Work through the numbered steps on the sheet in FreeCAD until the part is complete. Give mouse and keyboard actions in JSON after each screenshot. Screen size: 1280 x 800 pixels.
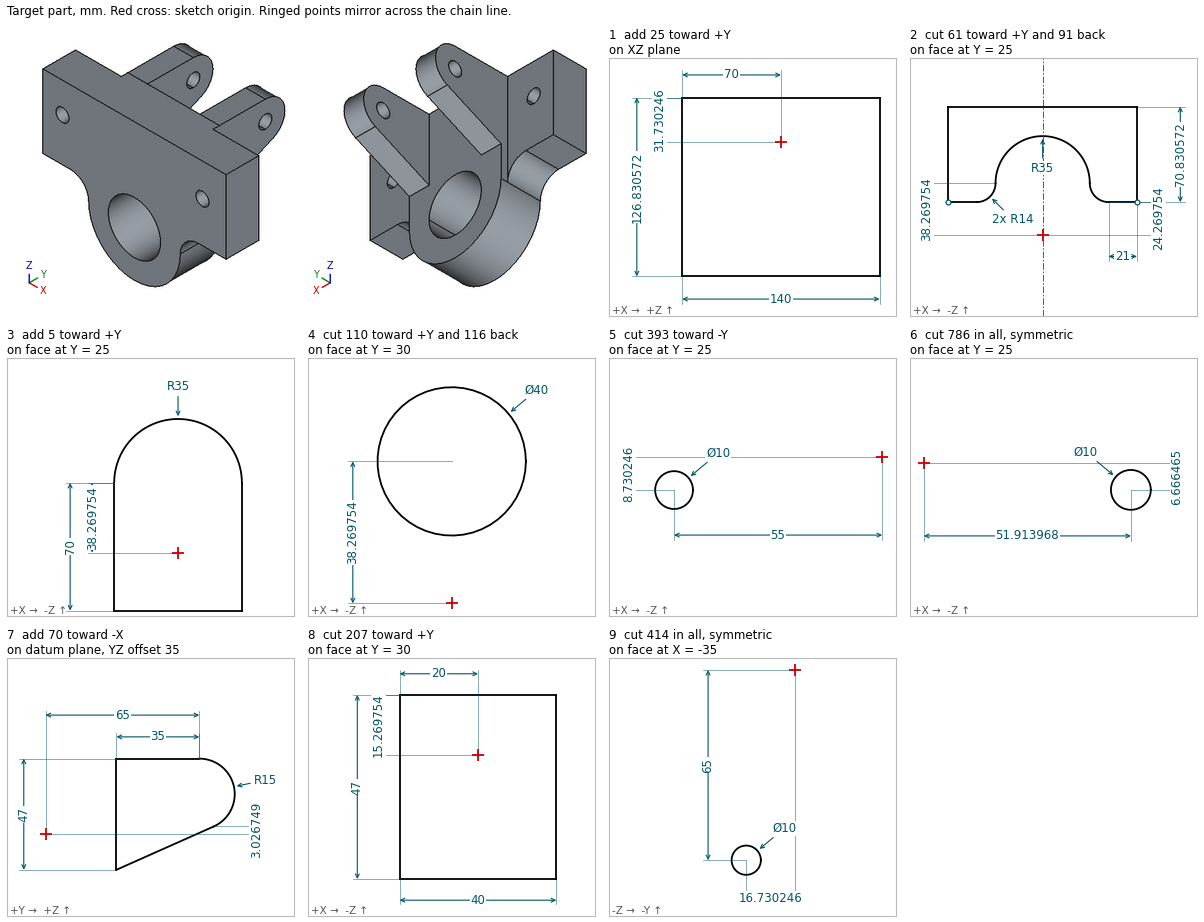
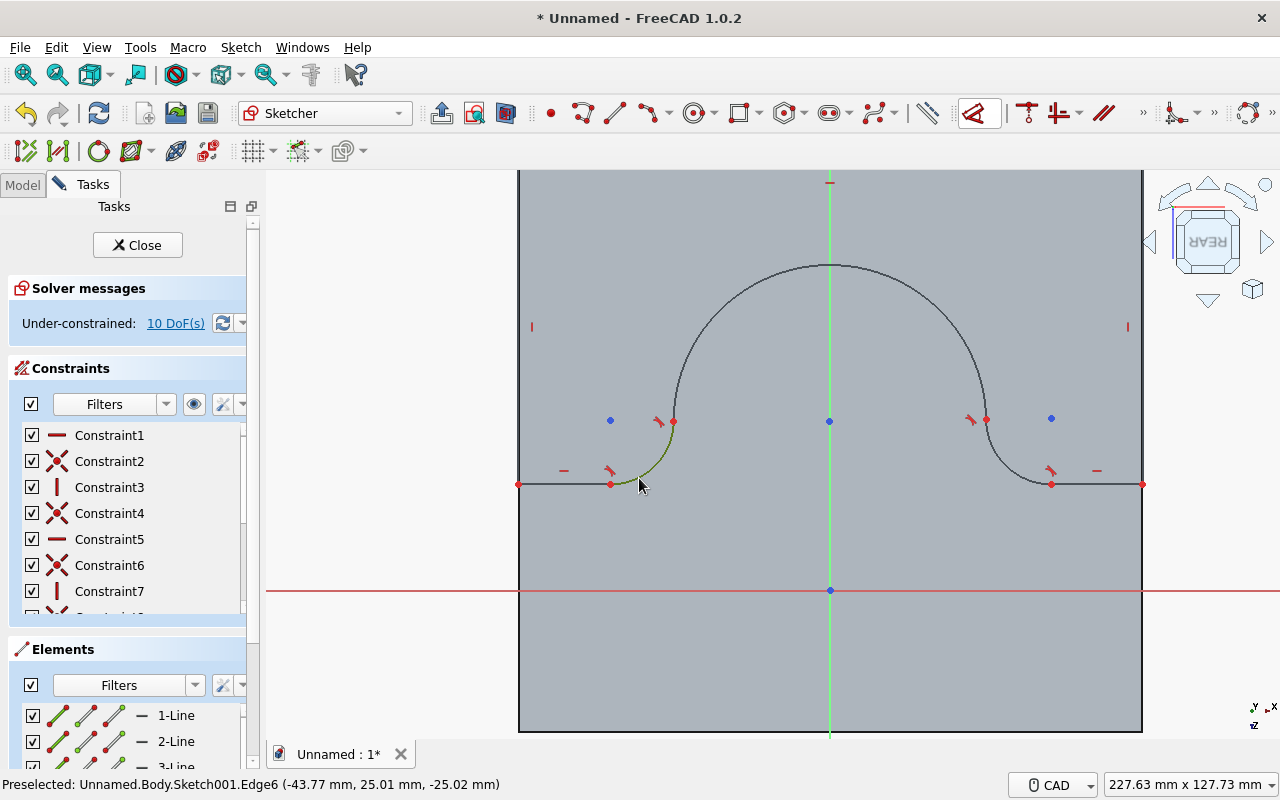
{"action": "left_click", "coordinate": [993, 449]}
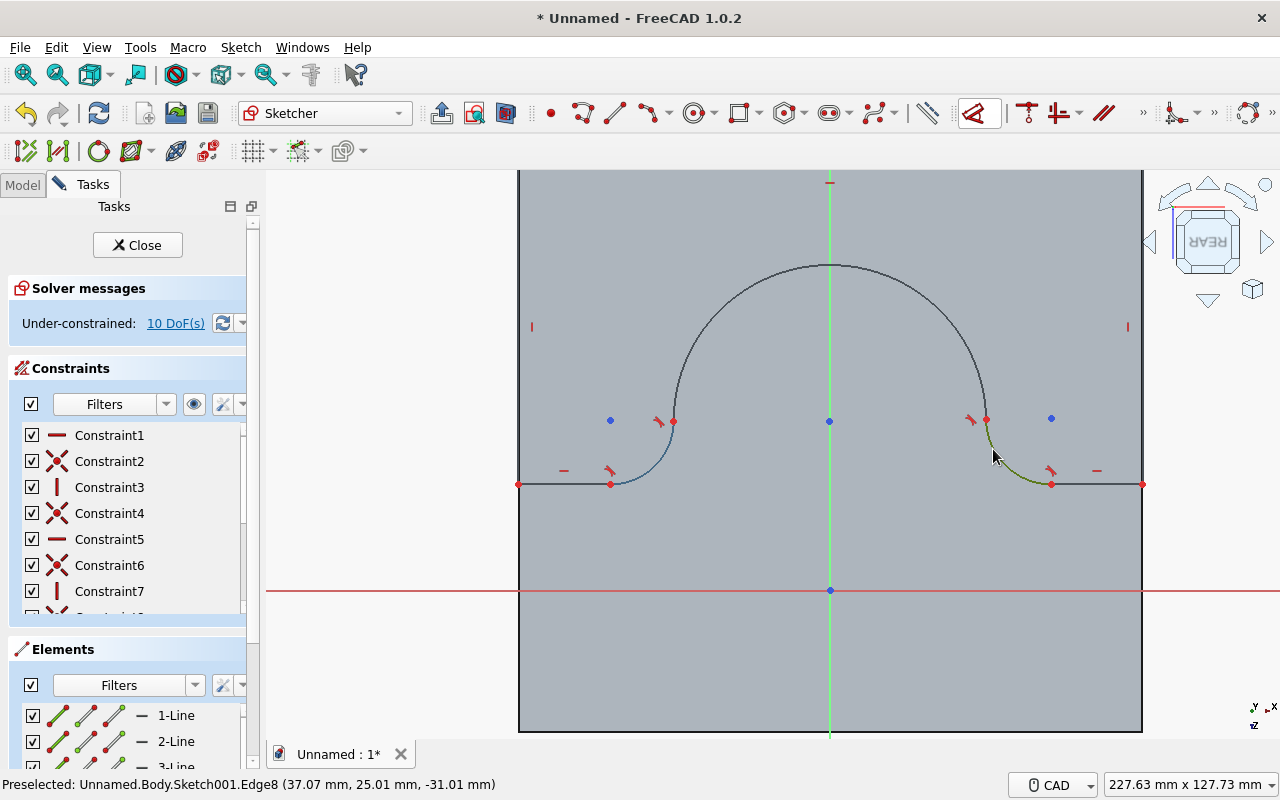
{"action": "key", "text": "e"}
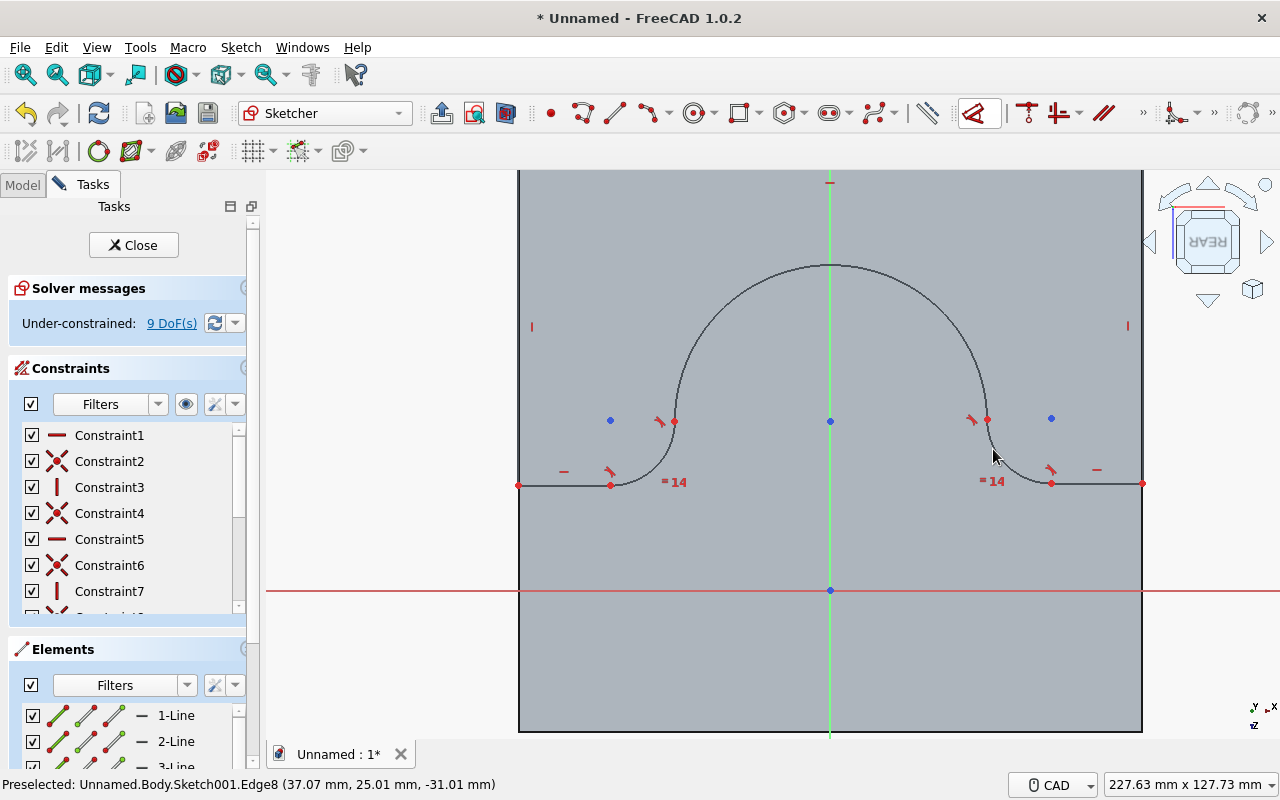
{"action": "left_click", "coordinate": [831, 421]}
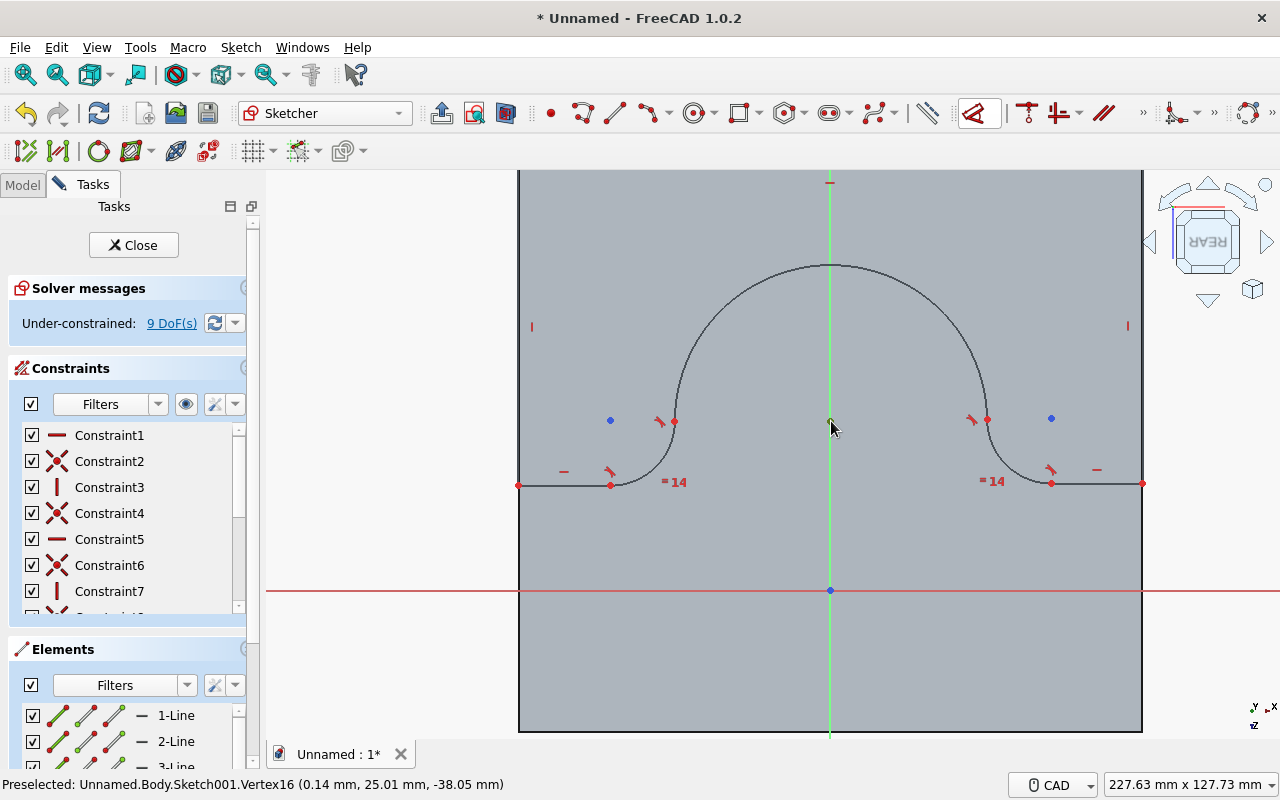
{"action": "left_click", "coordinate": [830, 674]}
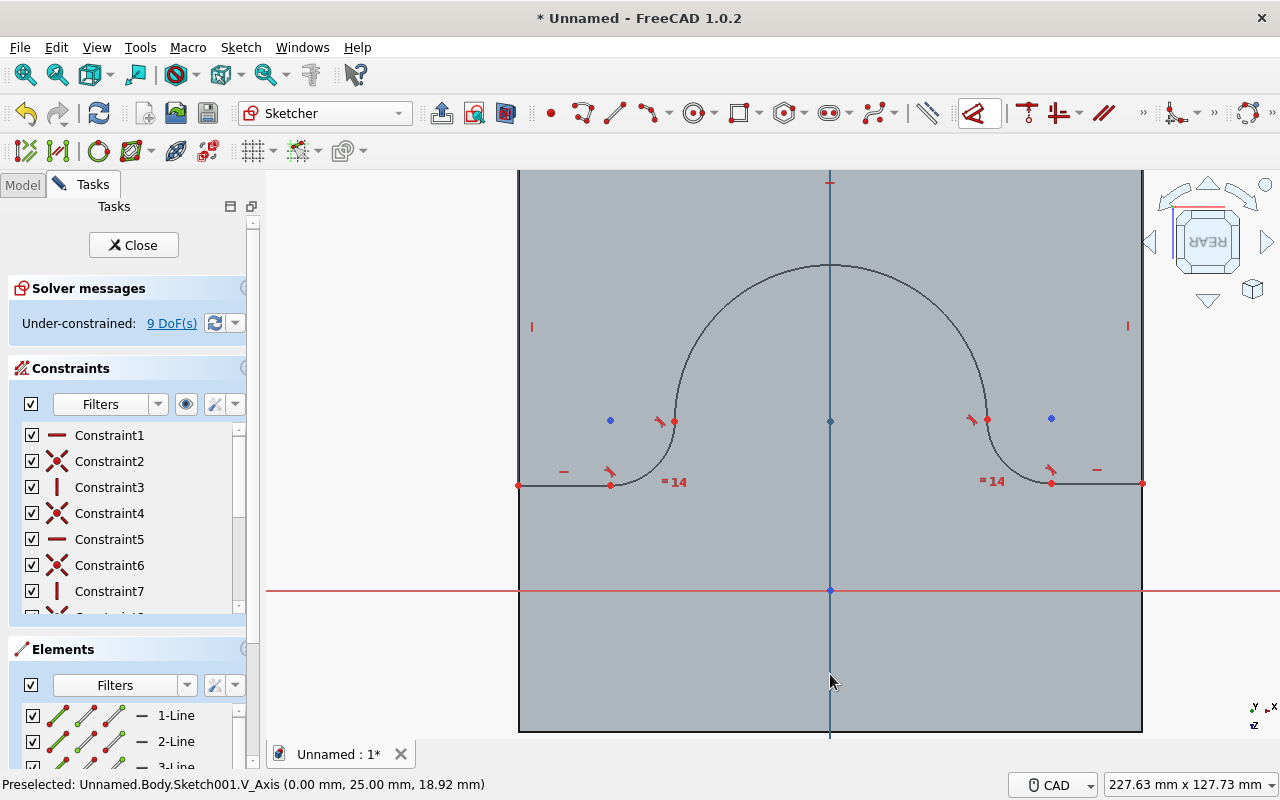
{"action": "left_click", "coordinate": [1028, 114]}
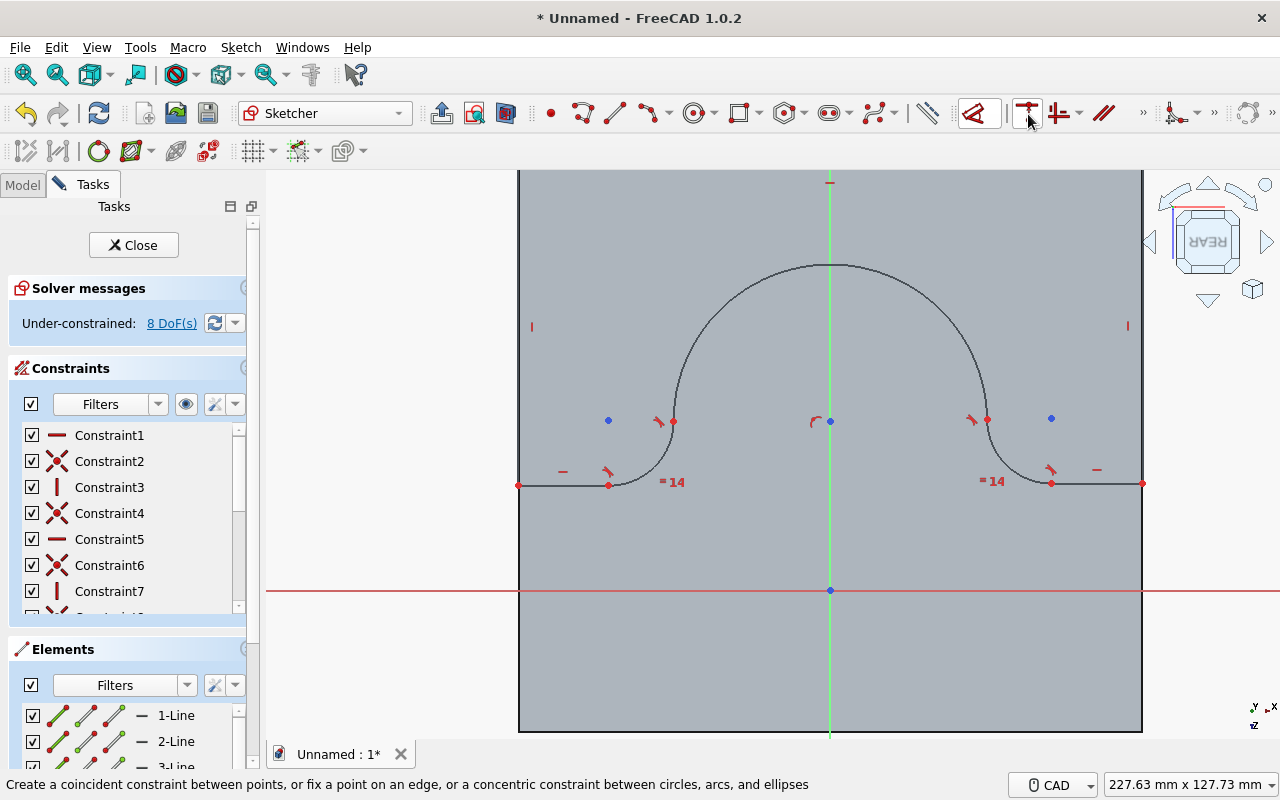
{"action": "scroll", "coordinate": [294, 711], "scroll_direction": "down", "scroll_amount": 1}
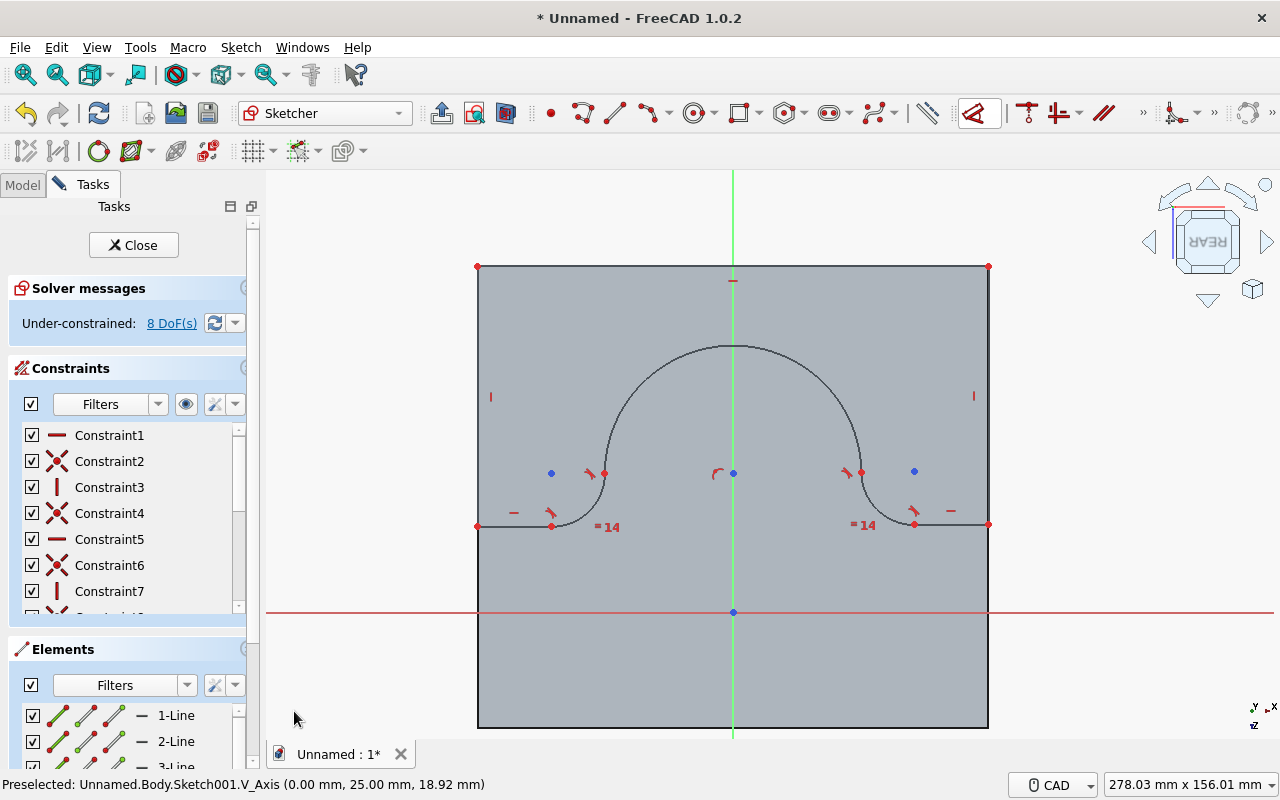
{"action": "left_click", "coordinate": [989, 525]}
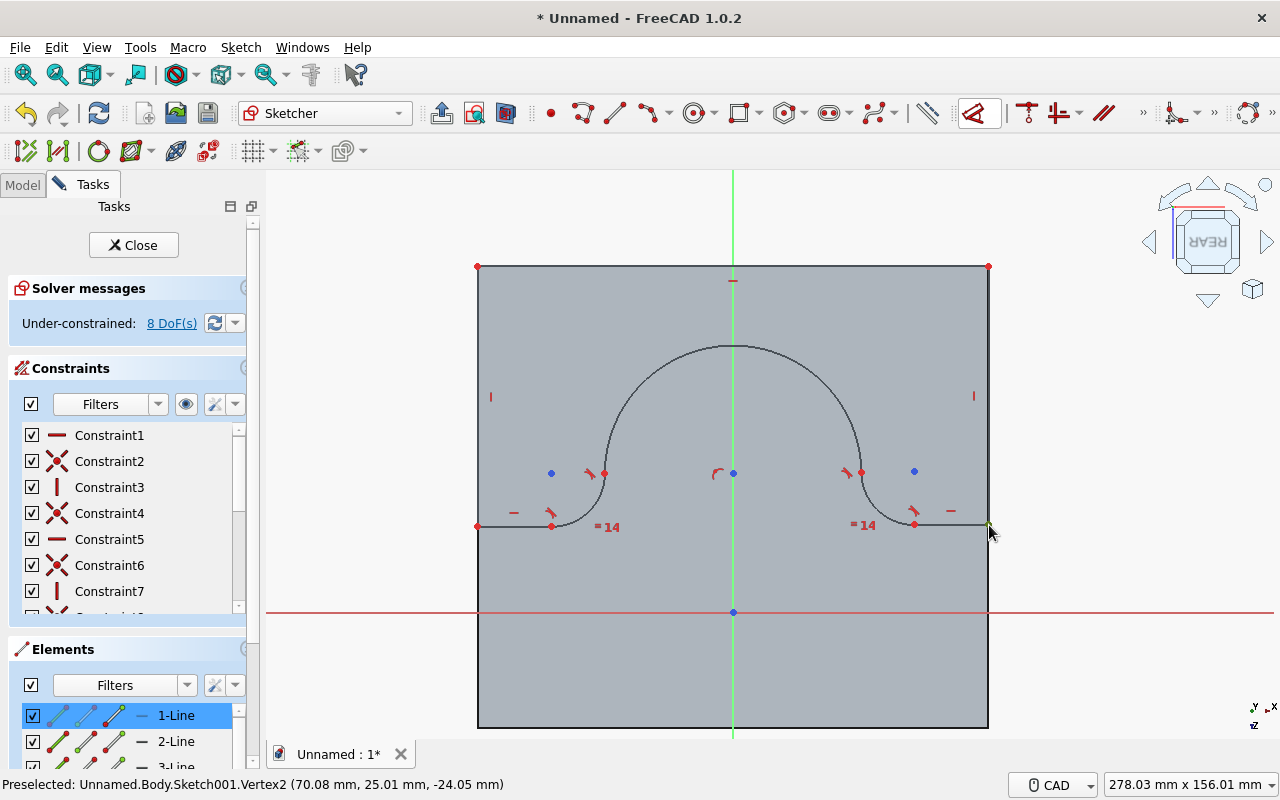
{"action": "left_click", "coordinate": [478, 527]}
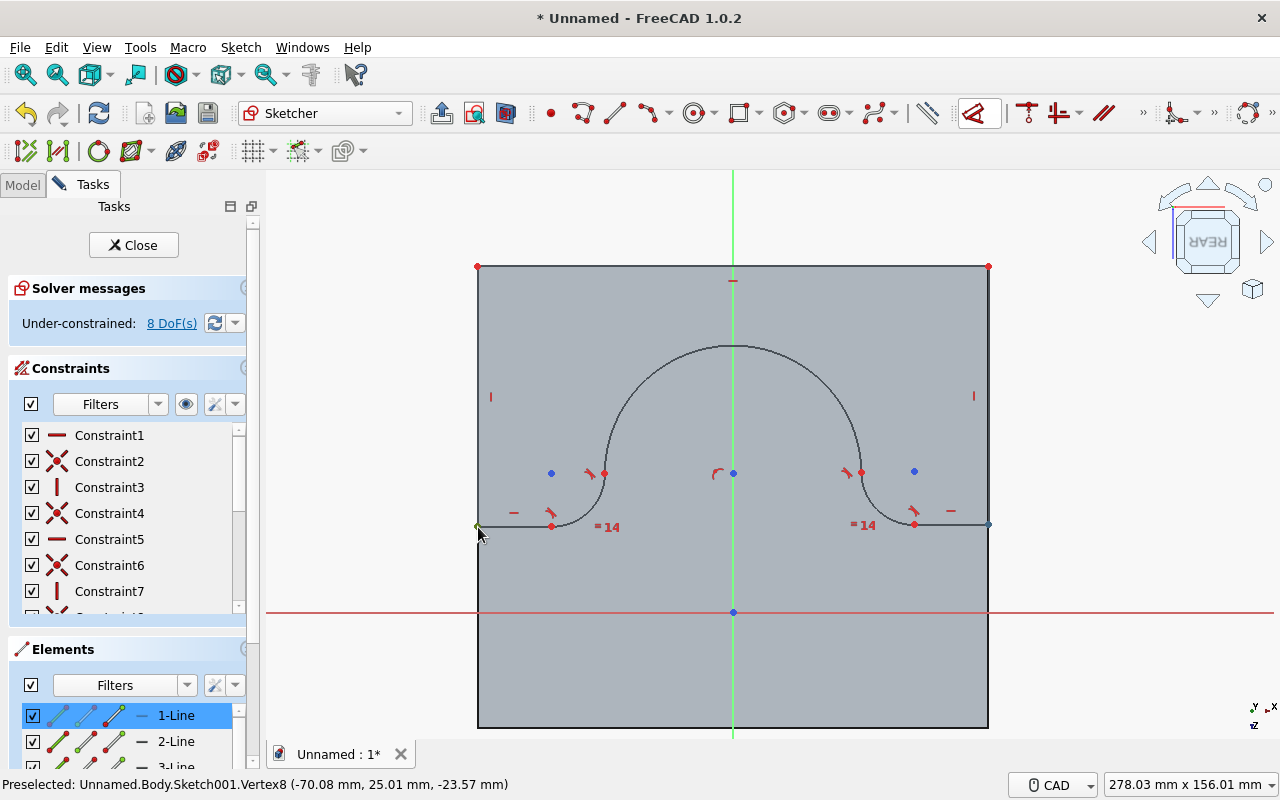
{"action": "left_click", "coordinate": [733, 674]}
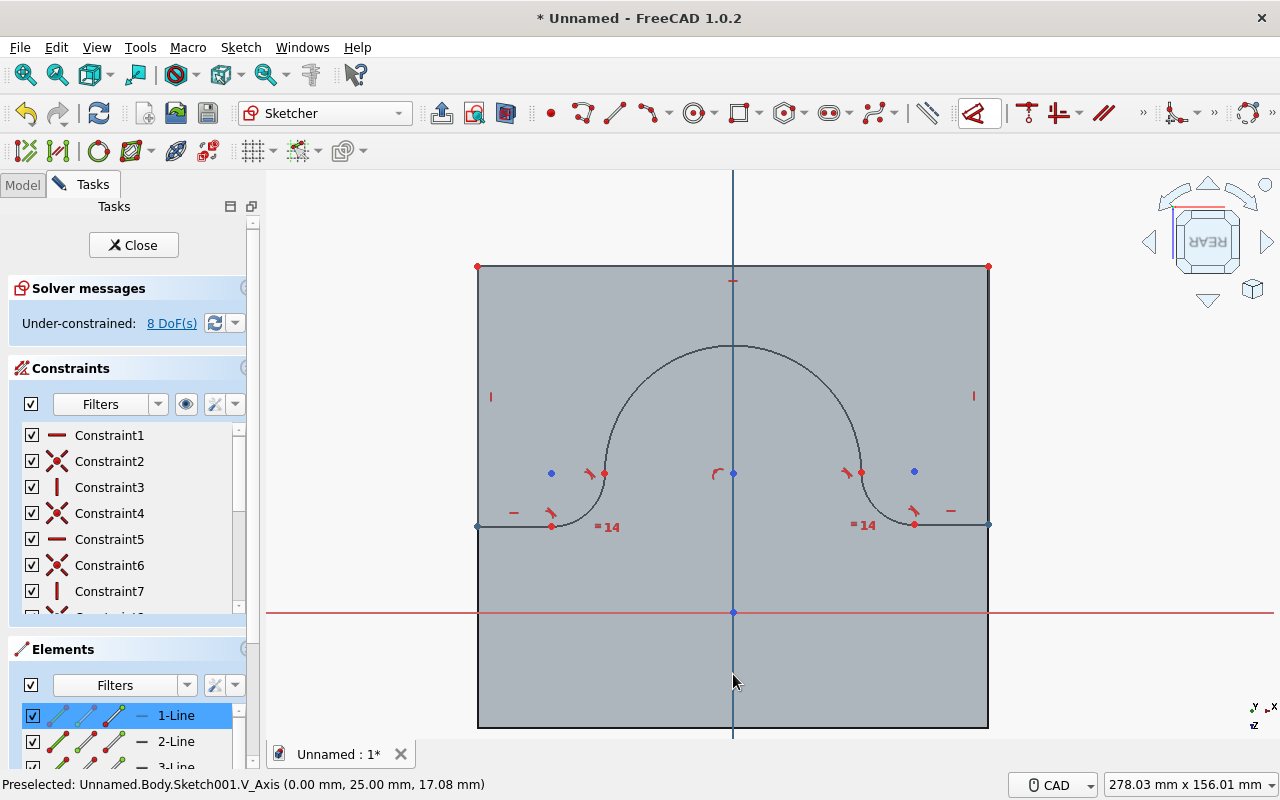
{"action": "key", "text": "s"}